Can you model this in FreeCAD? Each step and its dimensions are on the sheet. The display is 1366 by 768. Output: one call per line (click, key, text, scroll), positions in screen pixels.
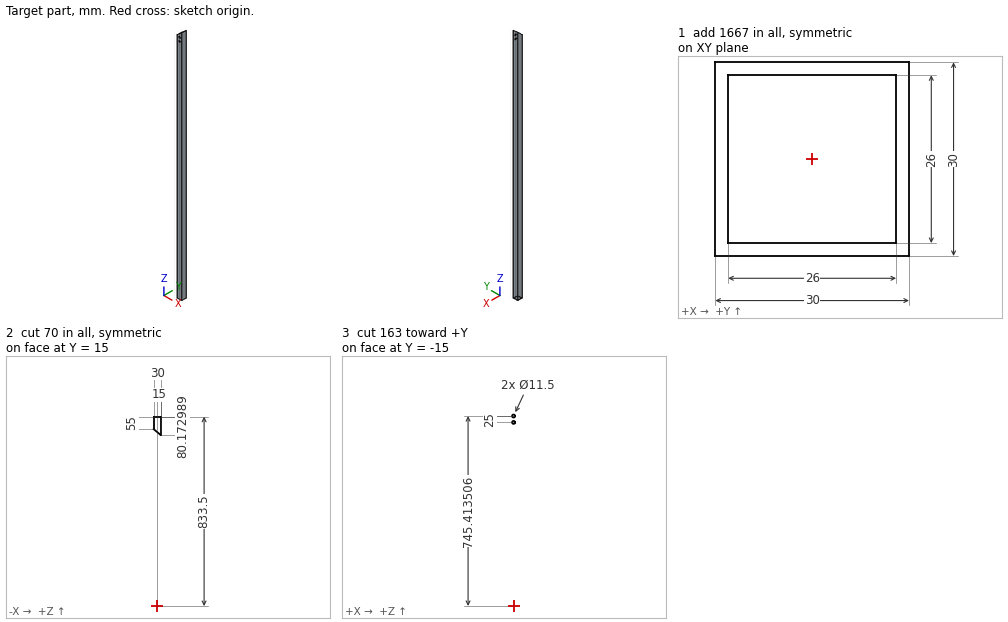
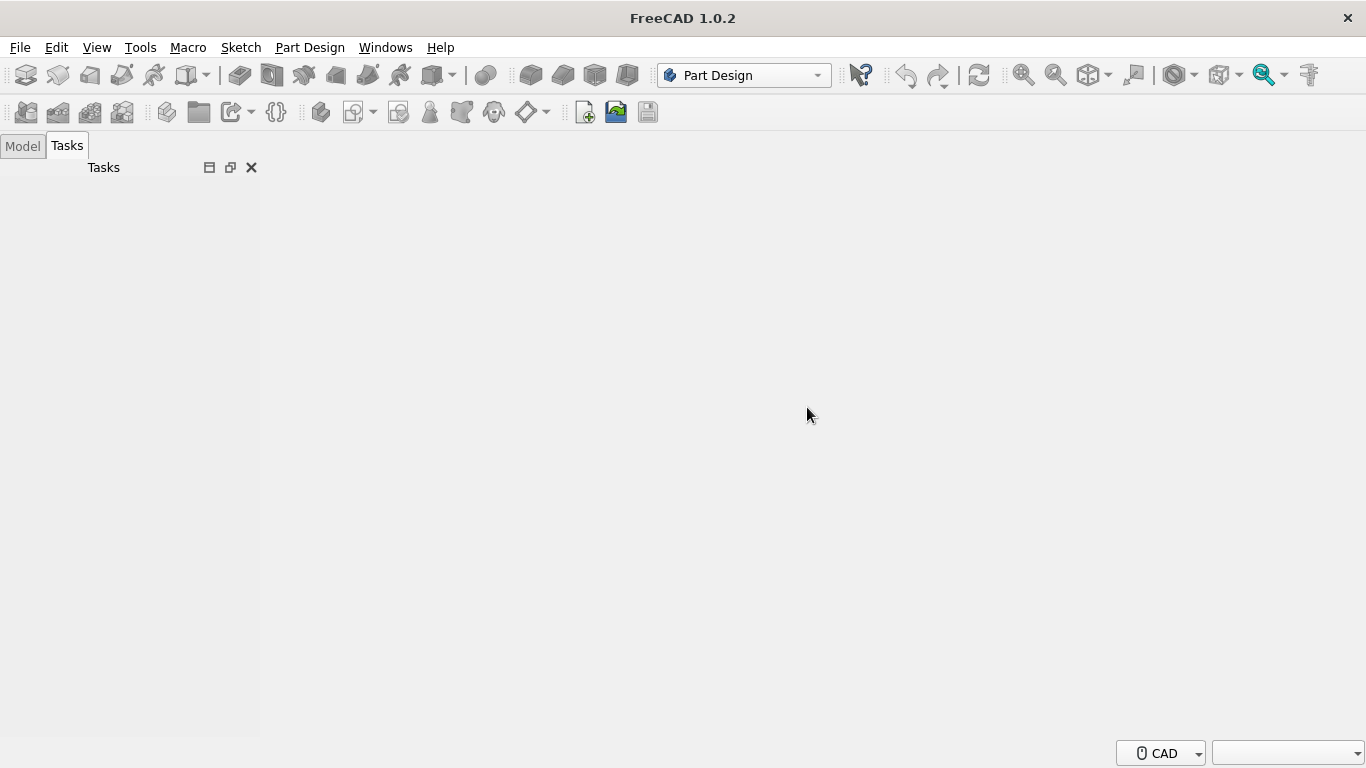
click(584, 112)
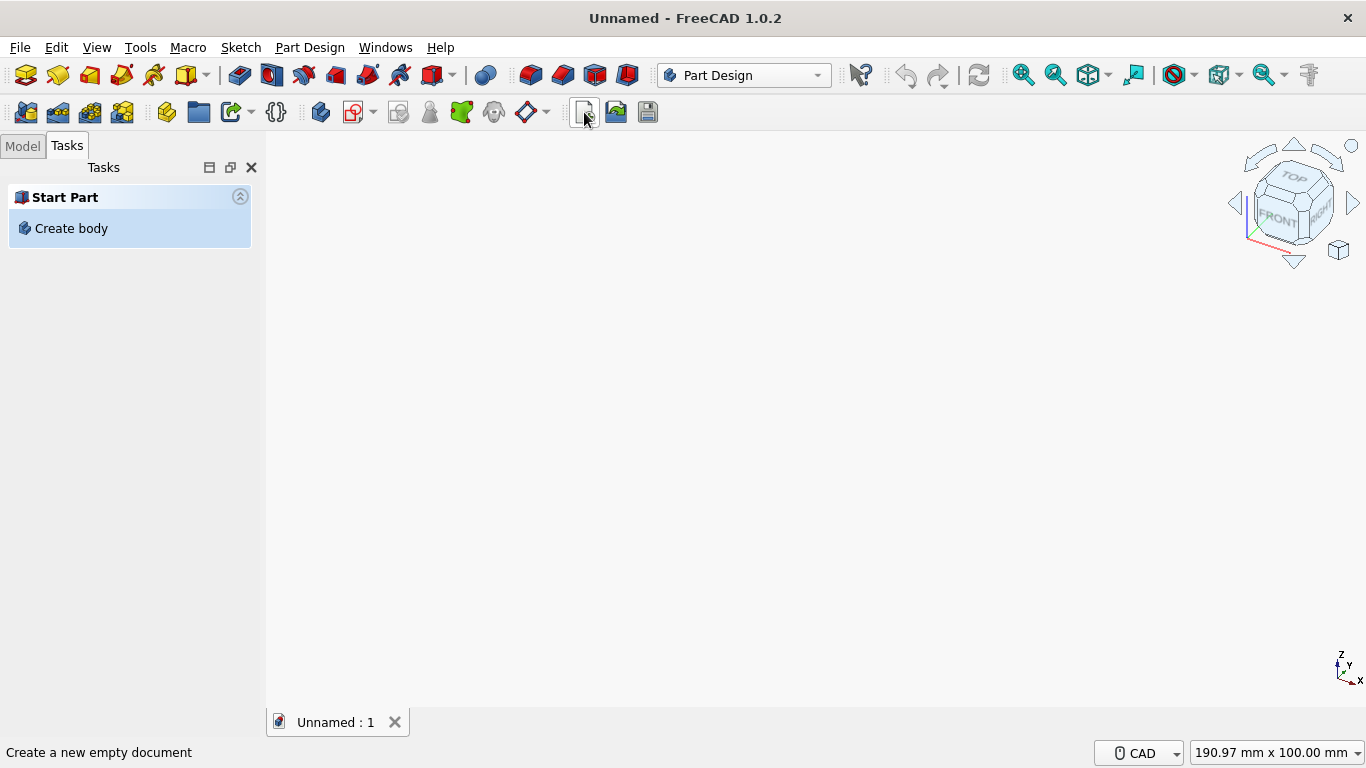
click(354, 112)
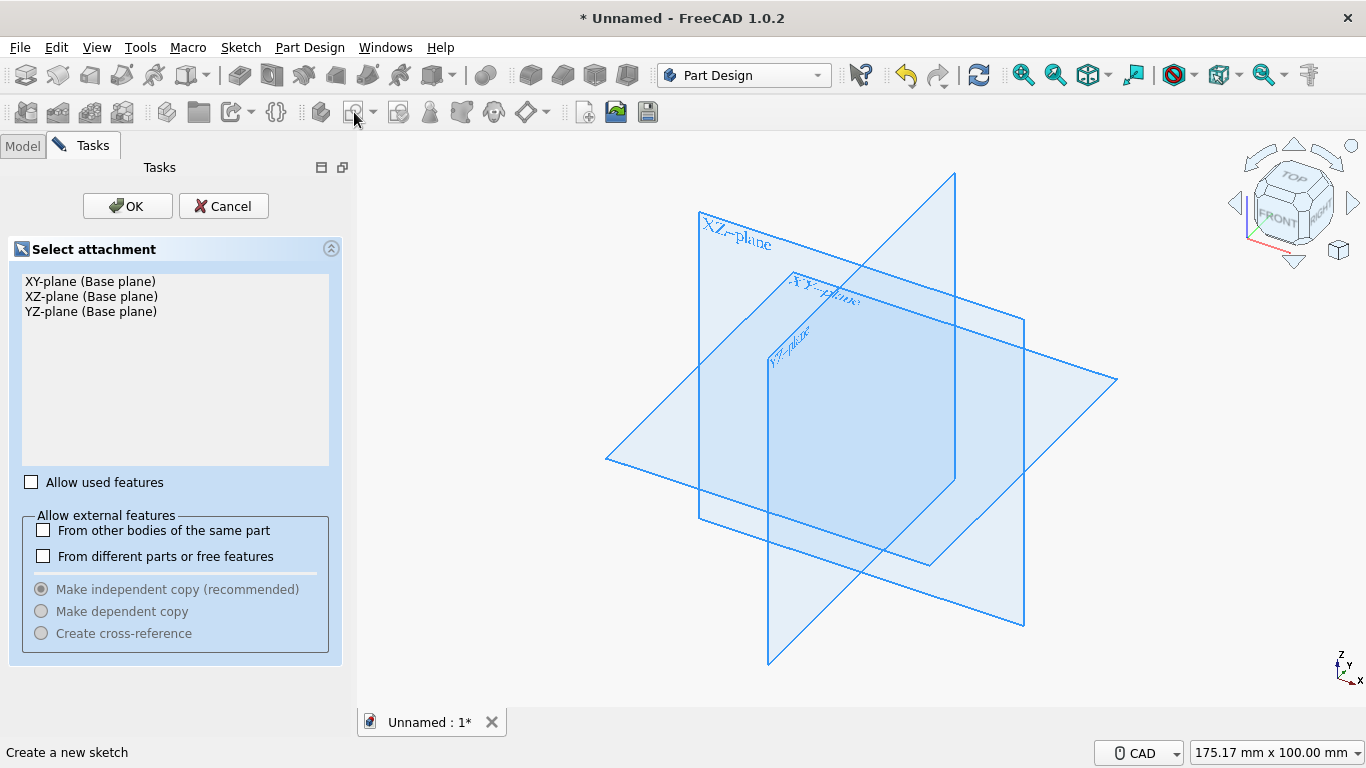
click(82, 282)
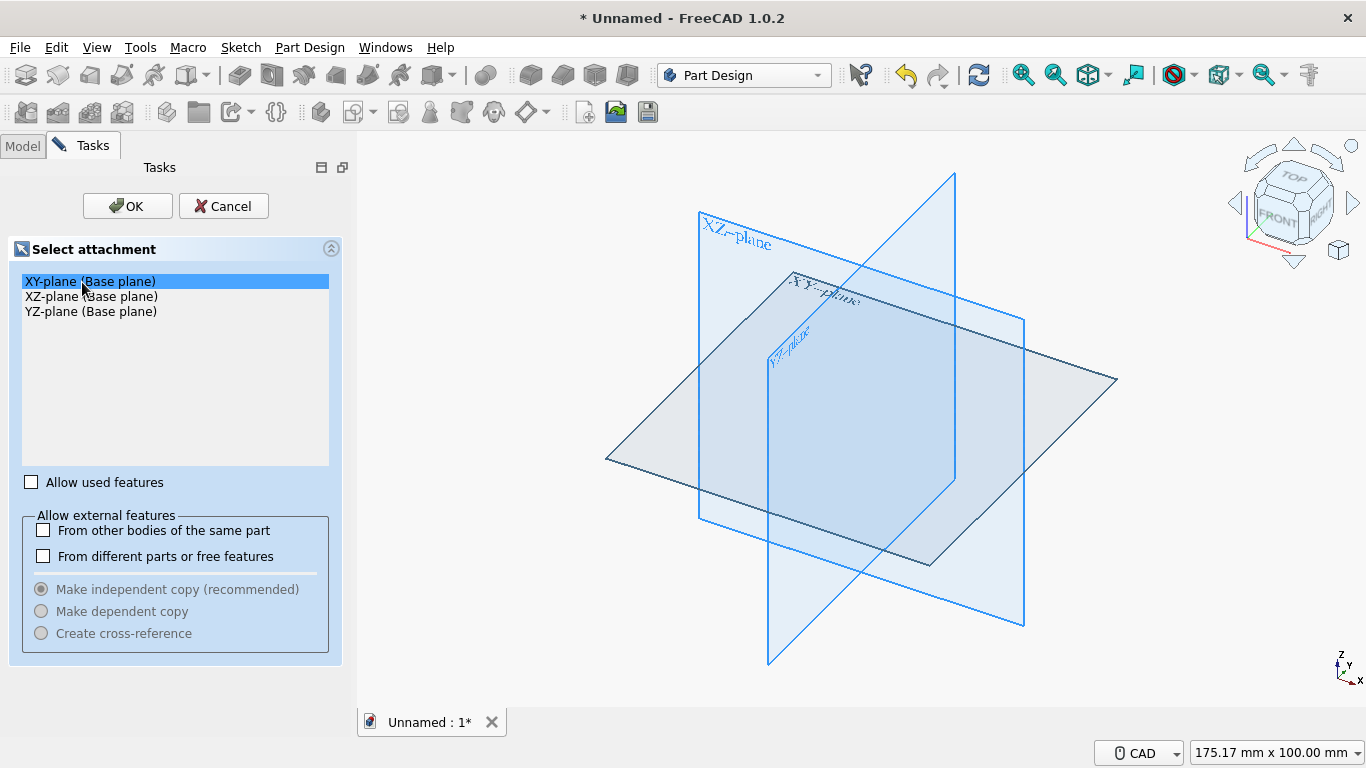
click(128, 206)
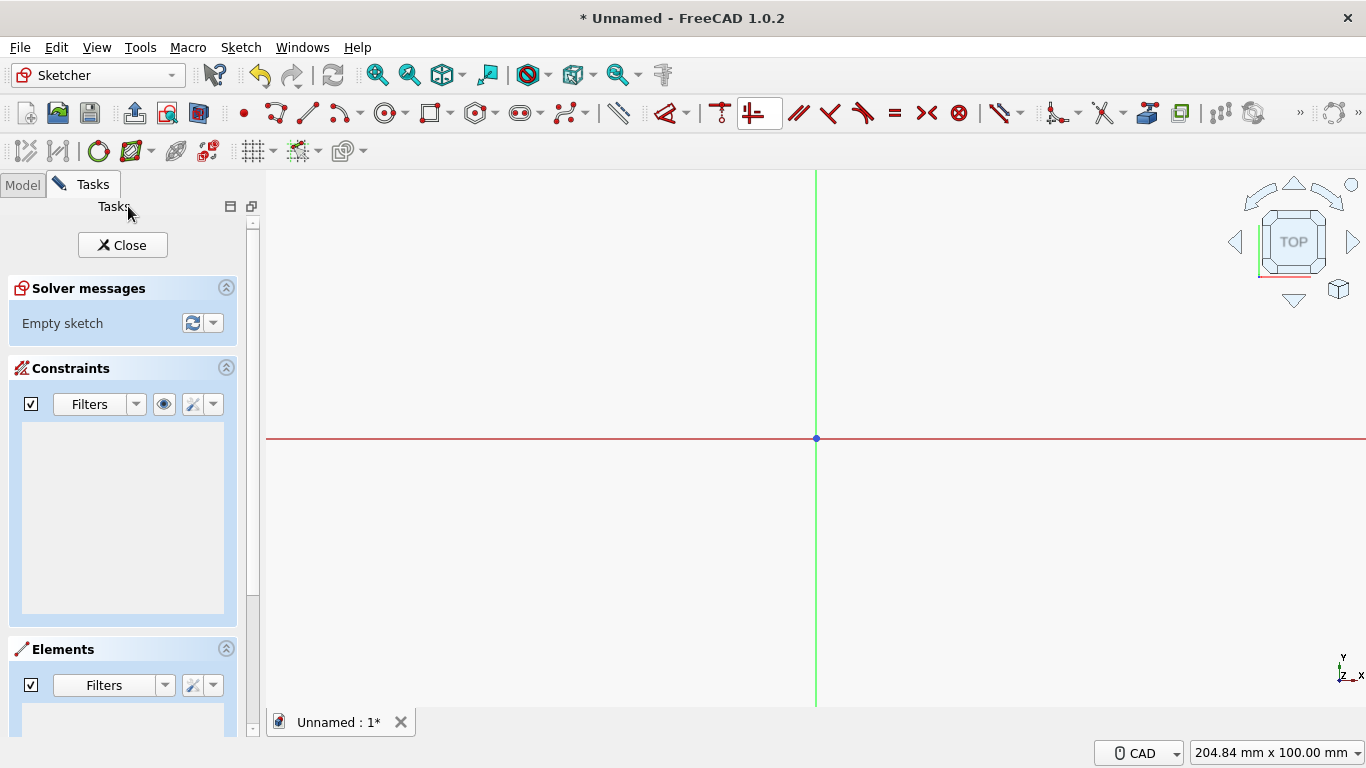
scroll(872, 438, up, 4)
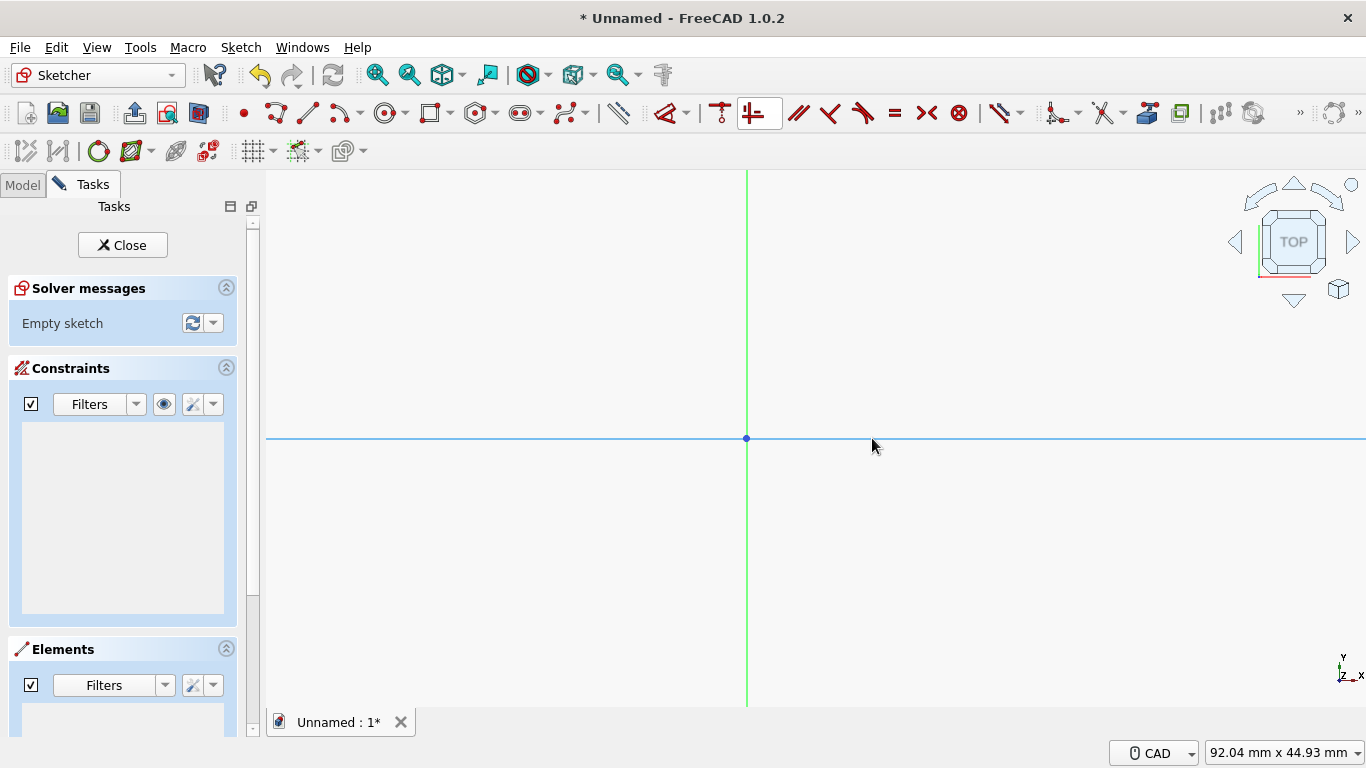
key(g)
key(v)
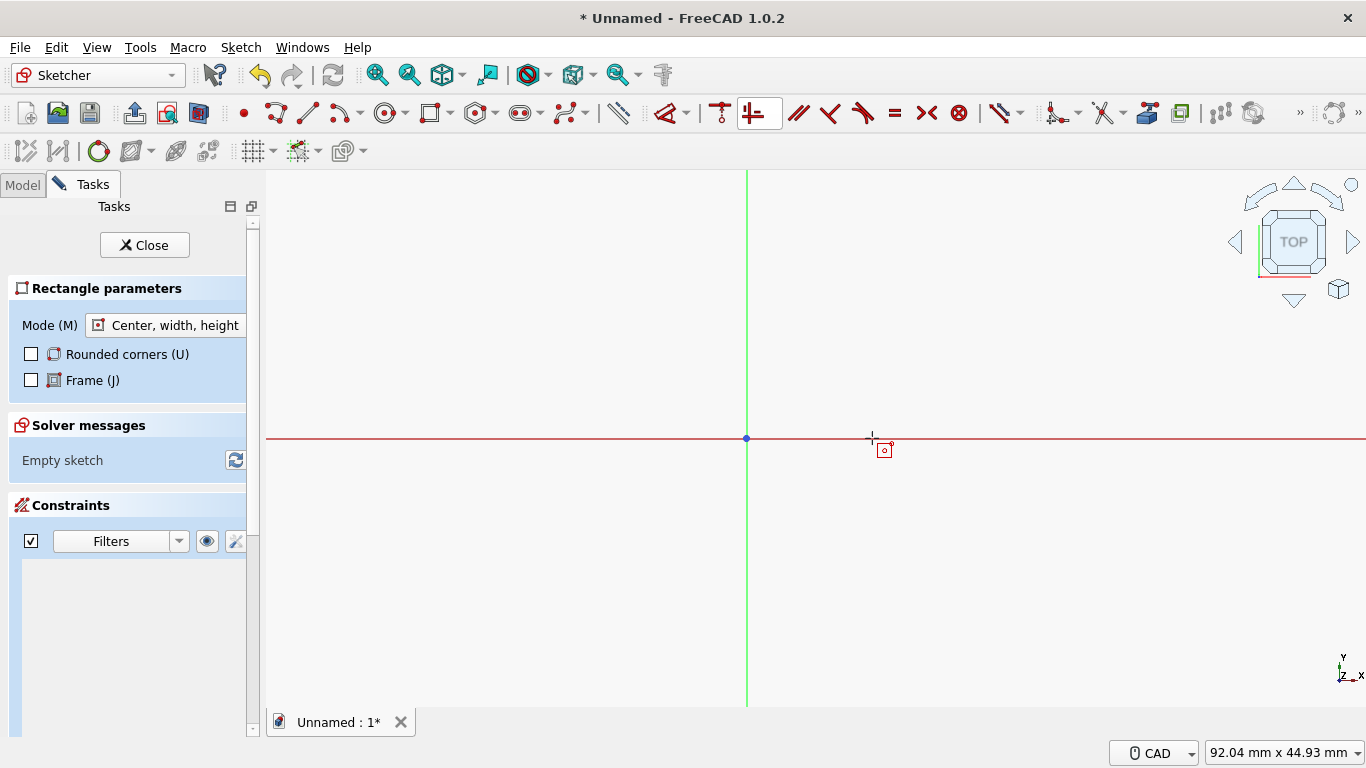
click(747, 438)
click(926, 259)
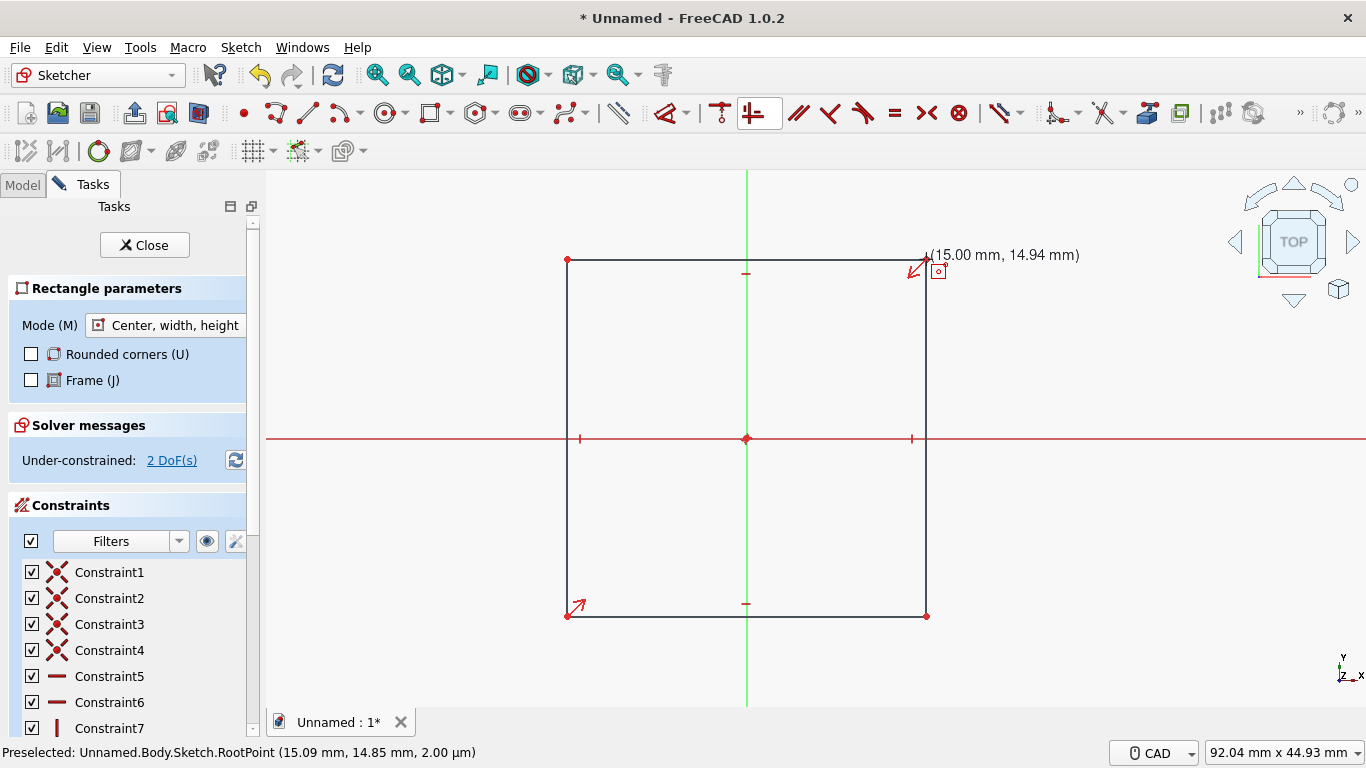
click(747, 438)
click(902, 283)
key(Escape)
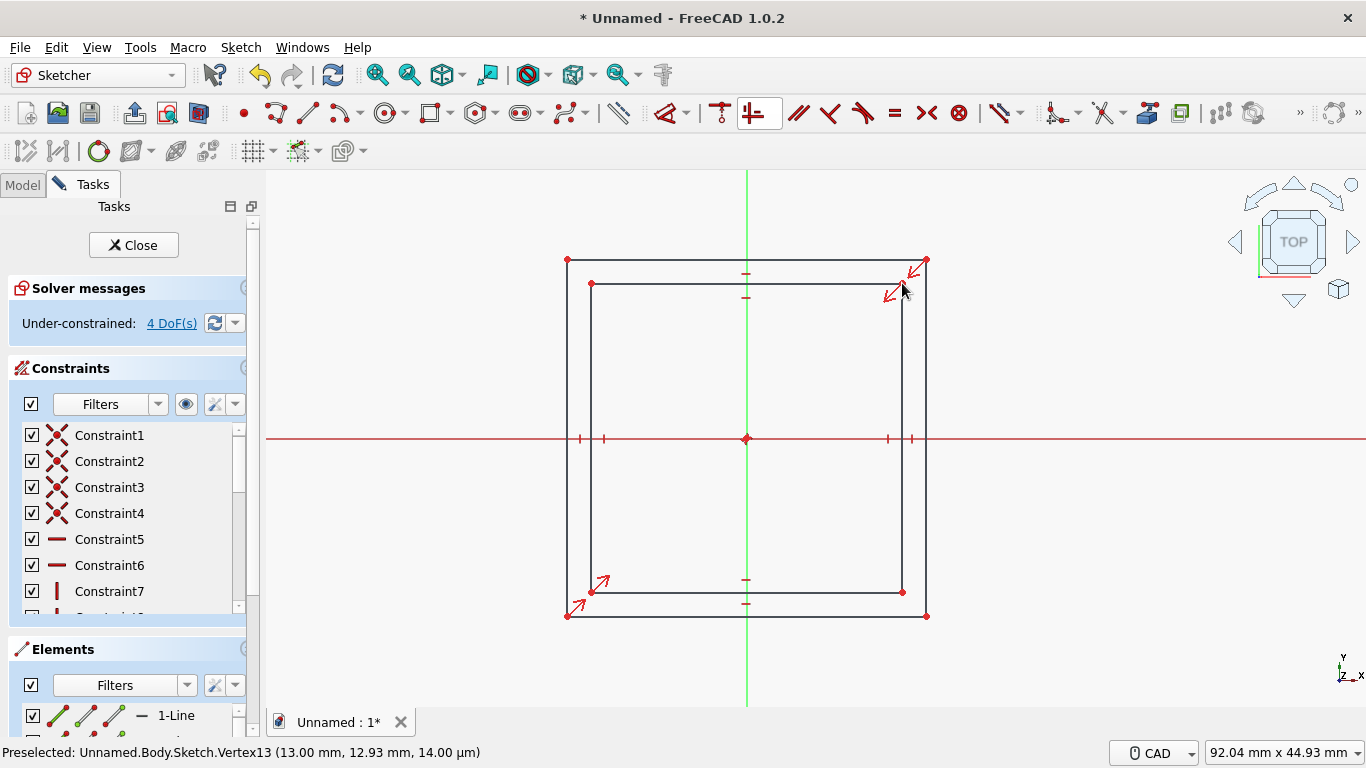
click(666, 114)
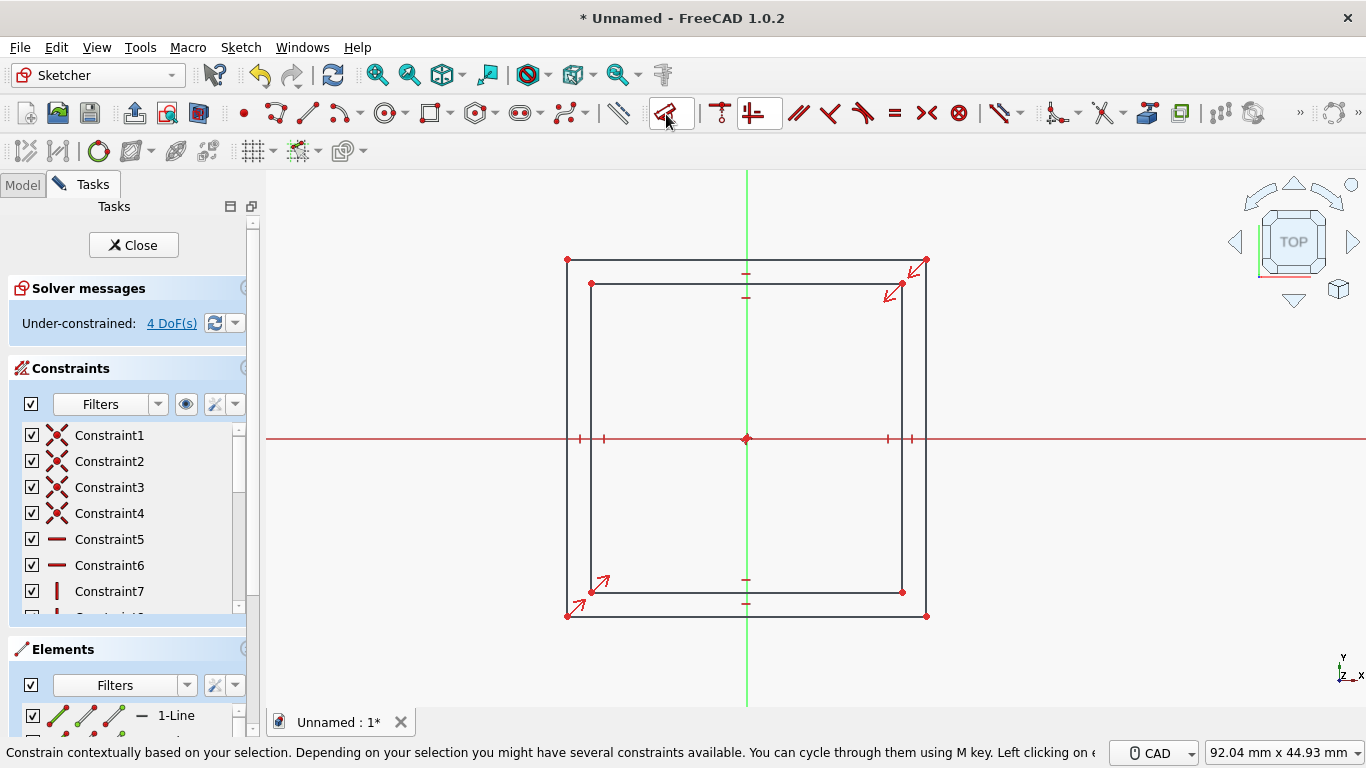
click(675, 617)
click(664, 651)